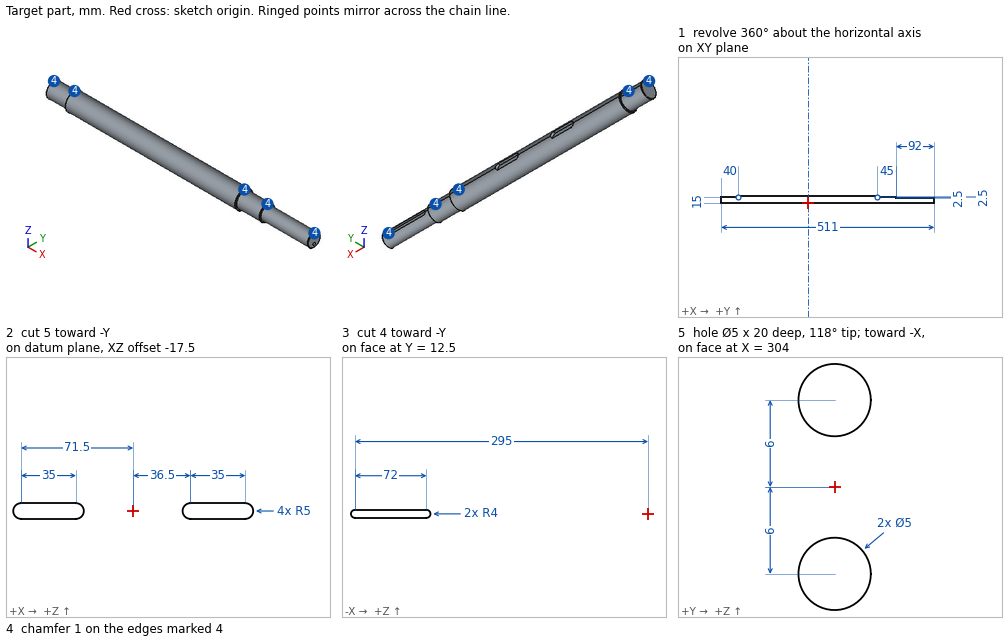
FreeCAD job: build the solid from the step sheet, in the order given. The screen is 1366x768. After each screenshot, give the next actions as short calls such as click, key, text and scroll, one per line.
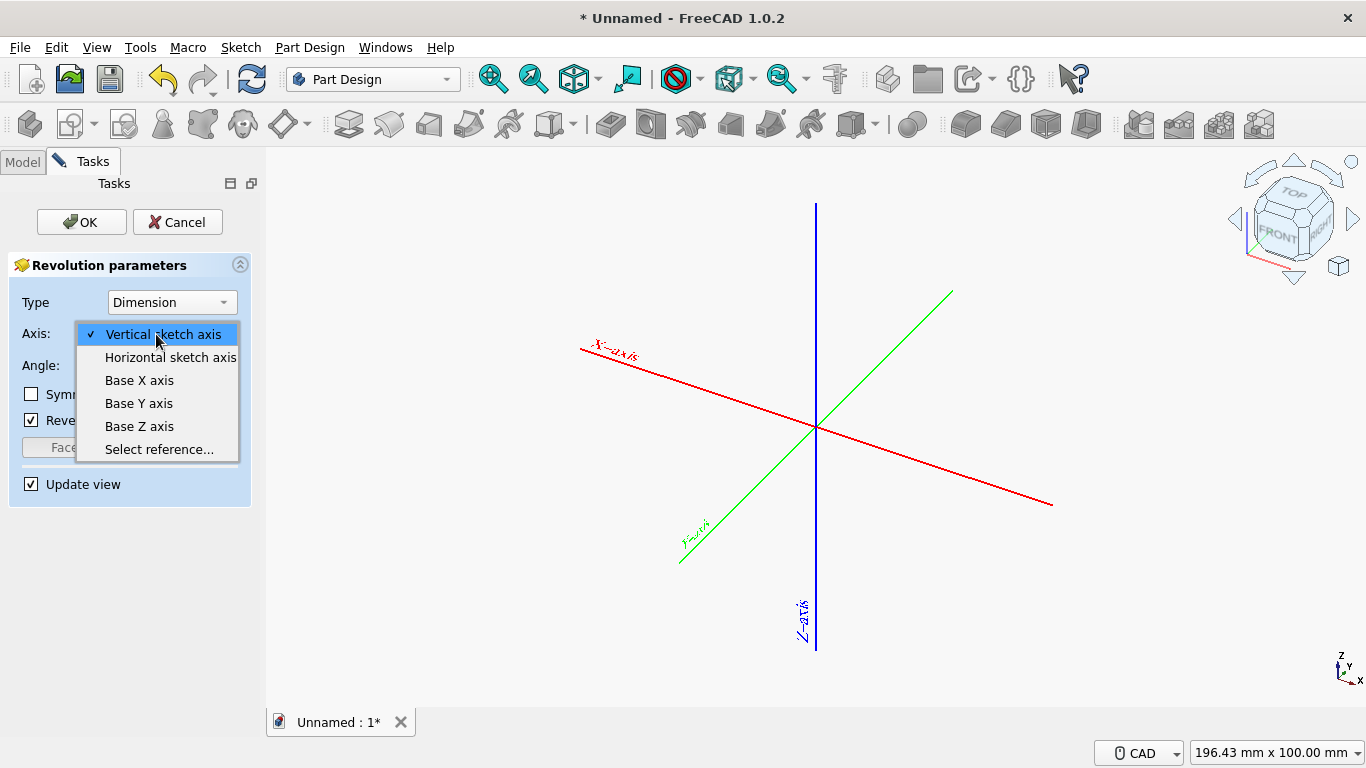
click(156, 358)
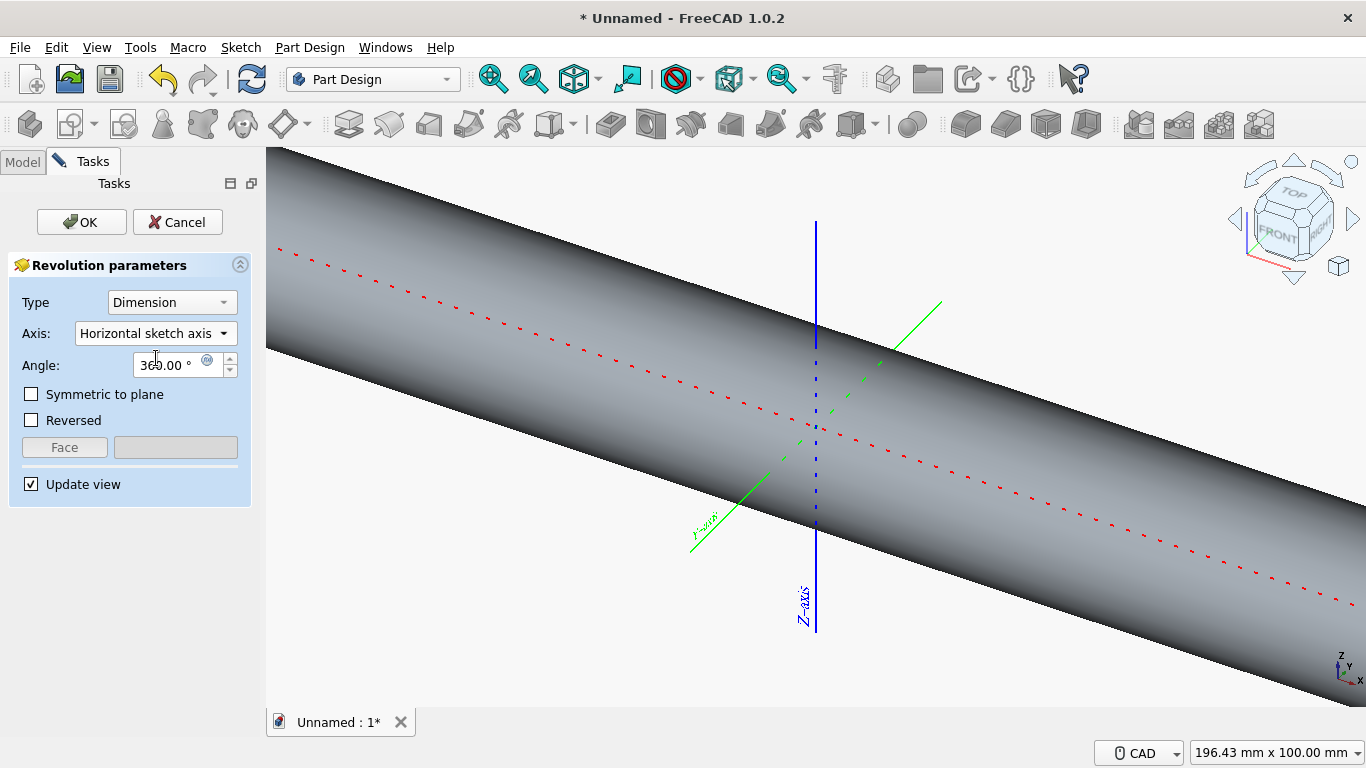
click(82, 222)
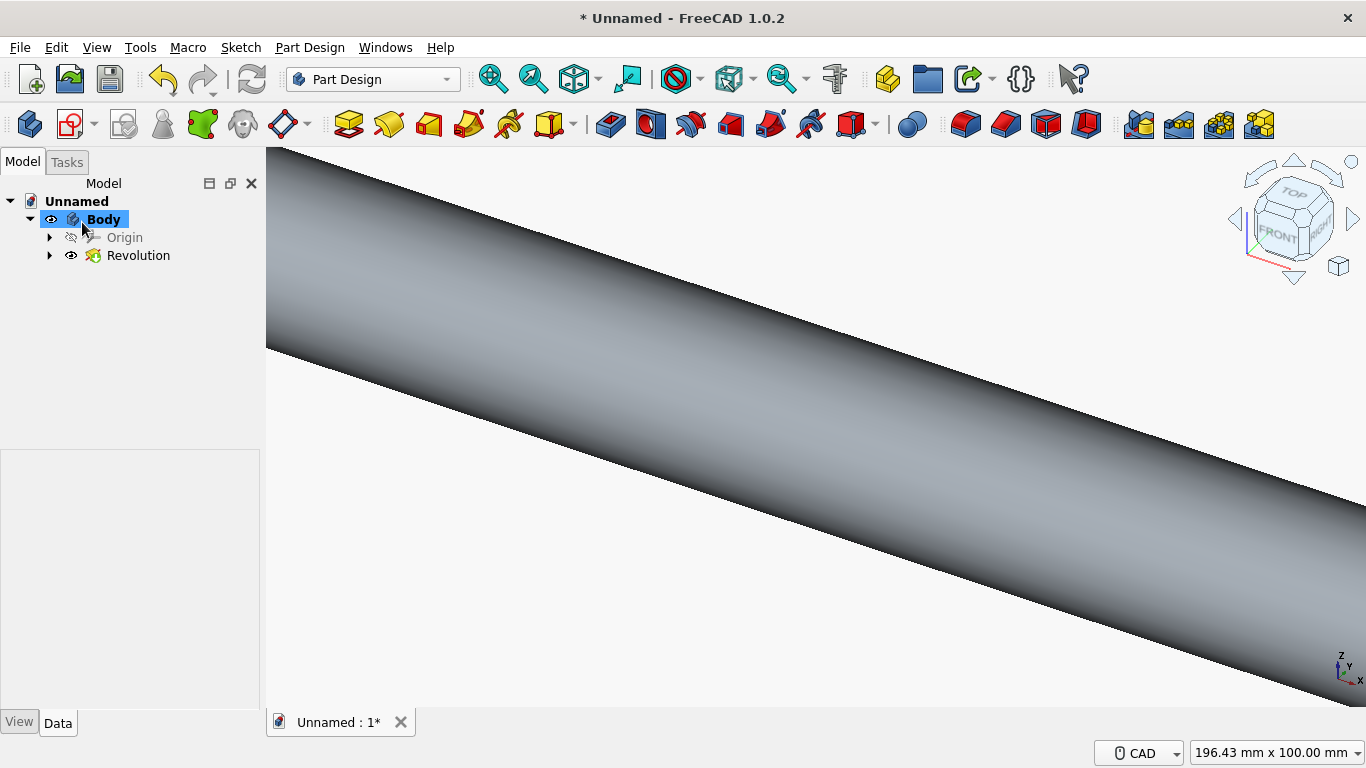
click(494, 80)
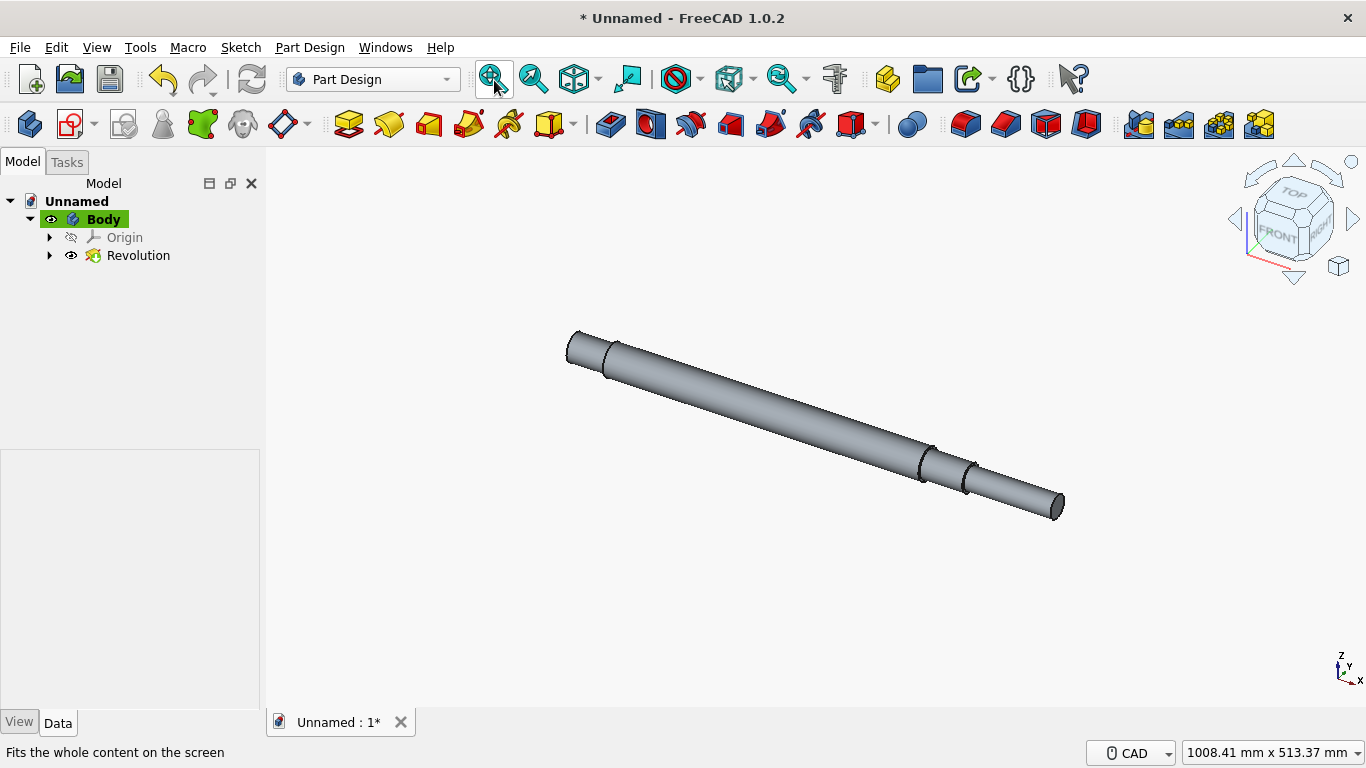
click(50, 237)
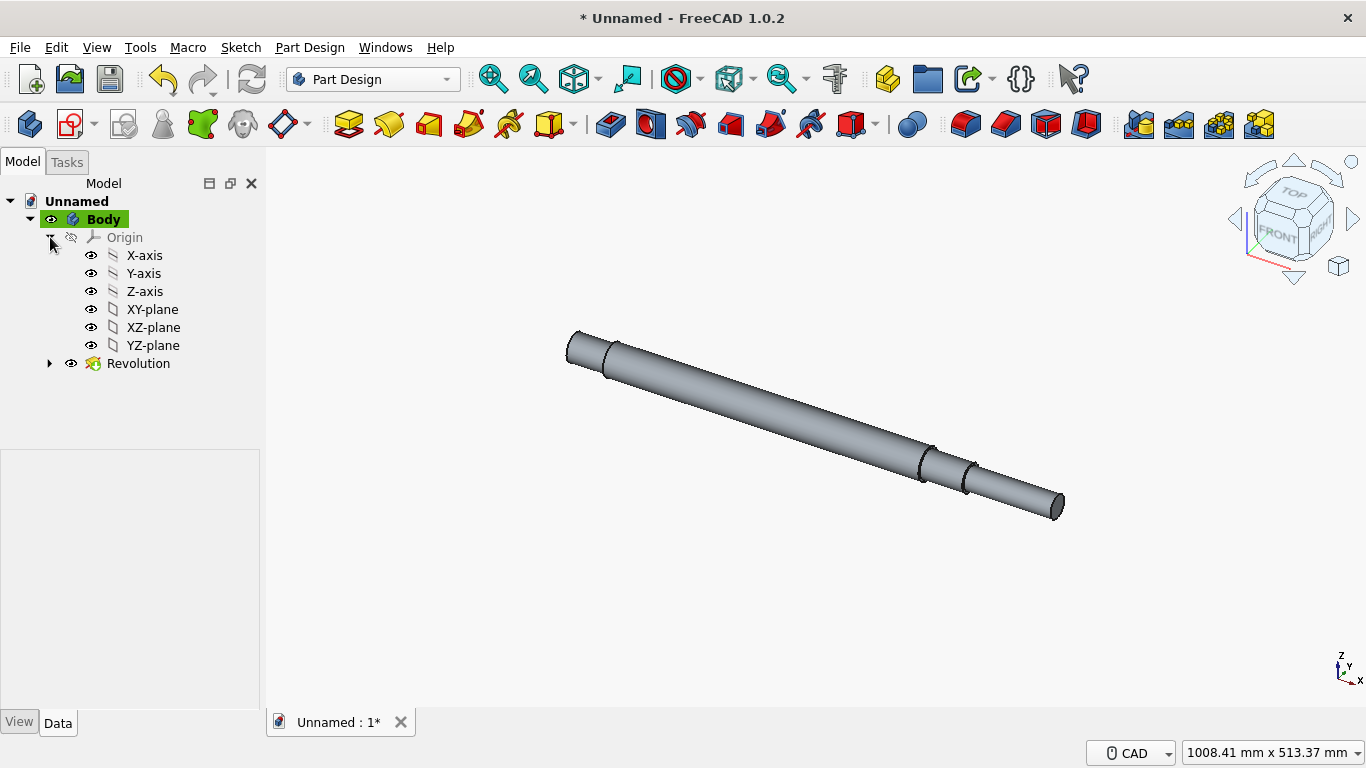
click(136, 327)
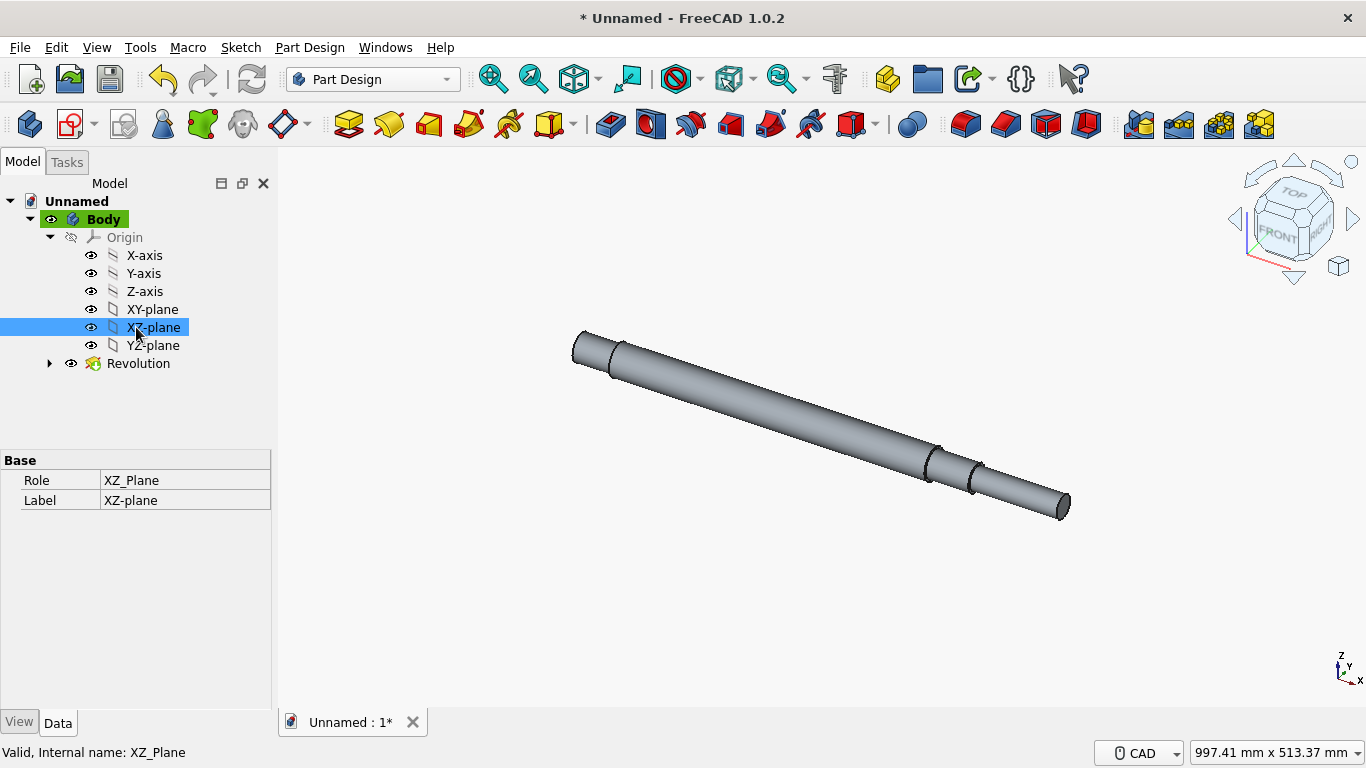
click(284, 124)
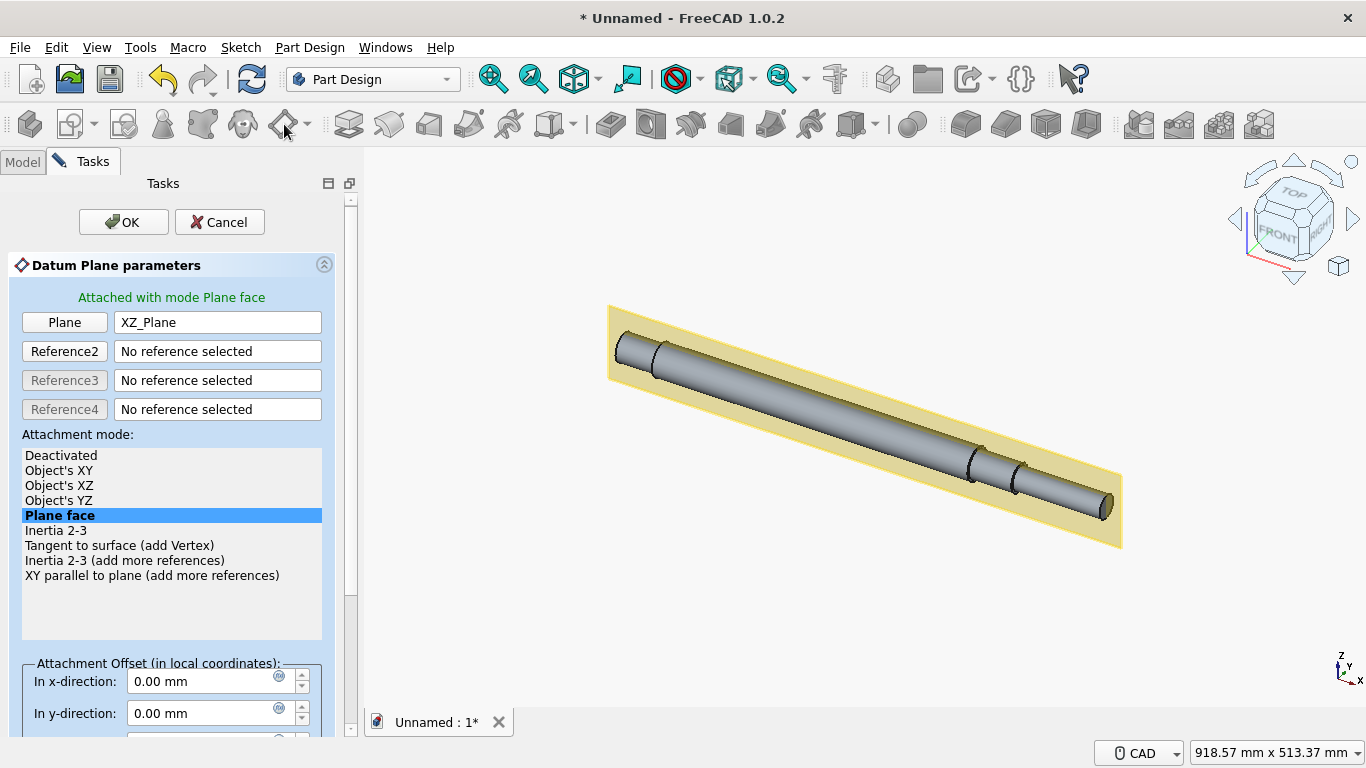
scroll(351, 464, down, 2)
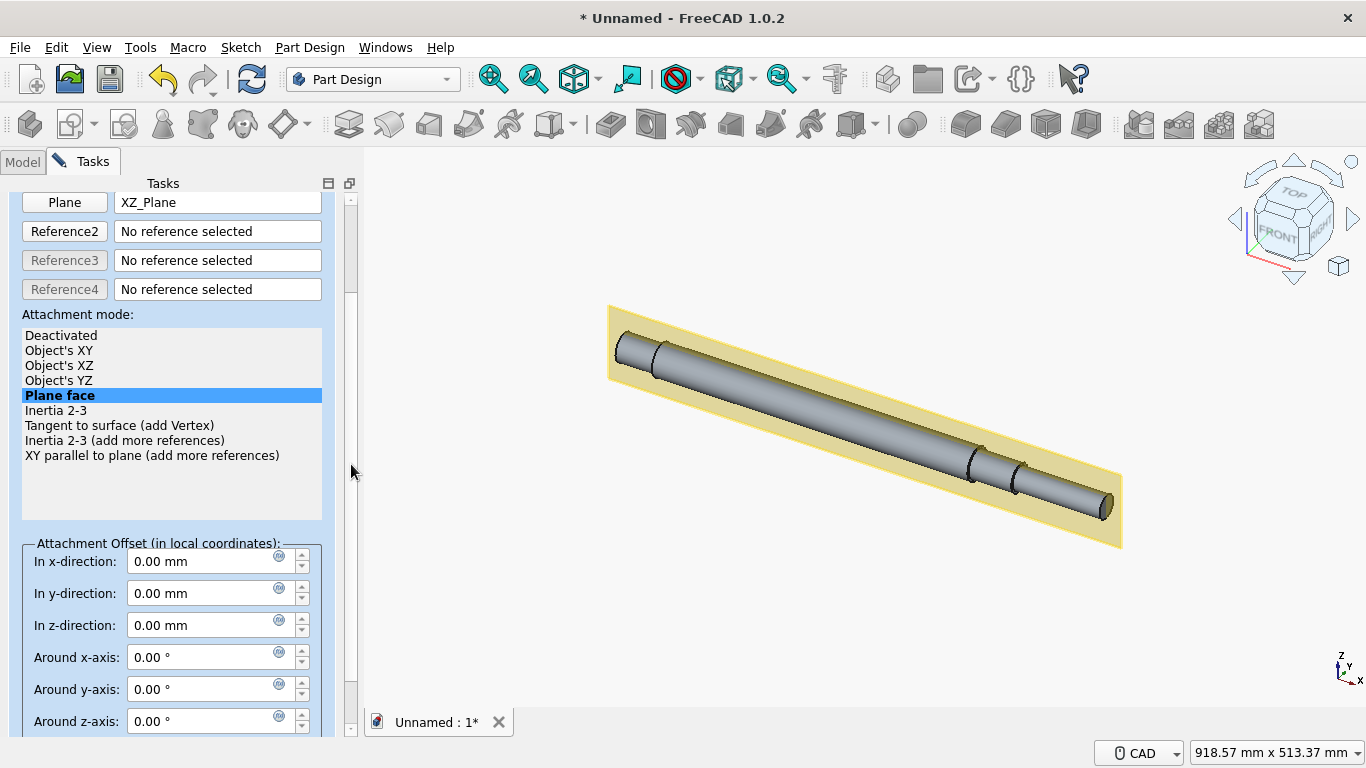
triple_click(210, 625)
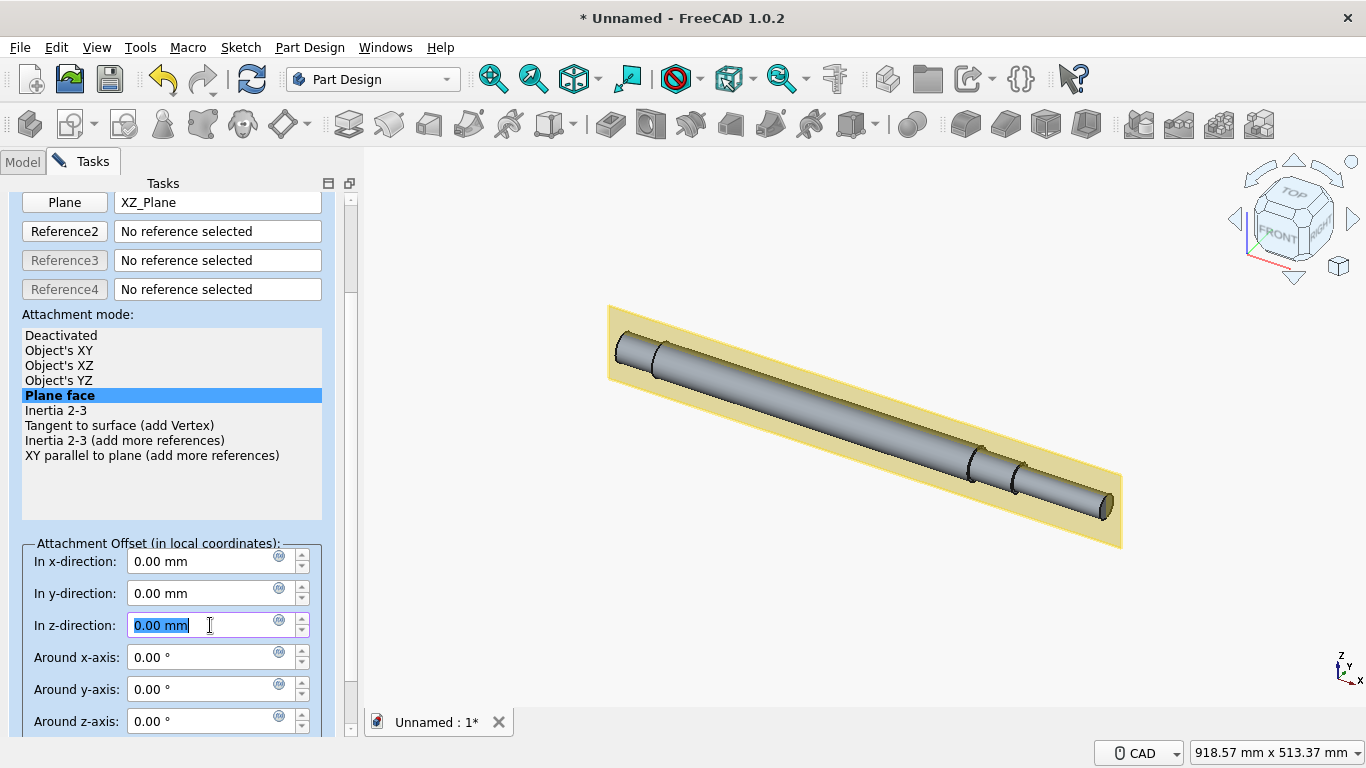
text(-17.5)
key(Tab)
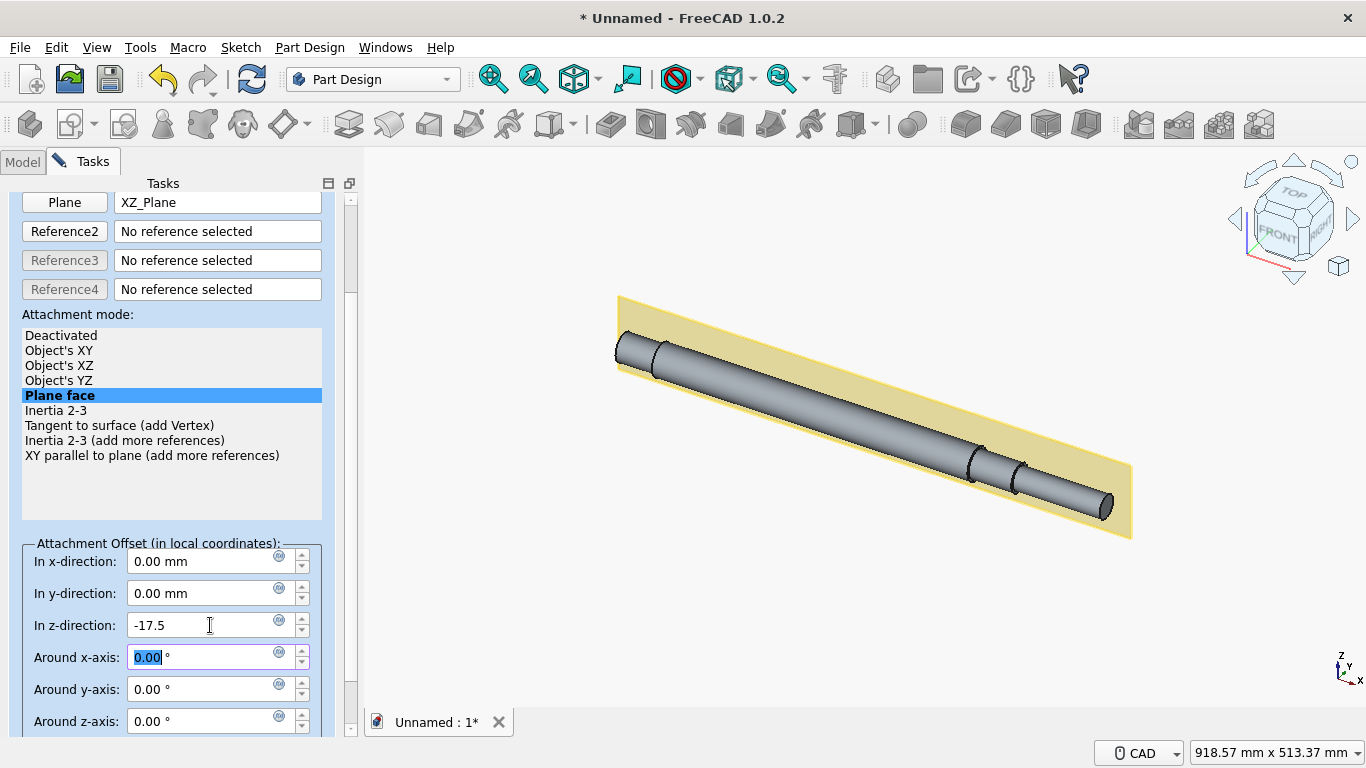
scroll(351, 464, up, 3)